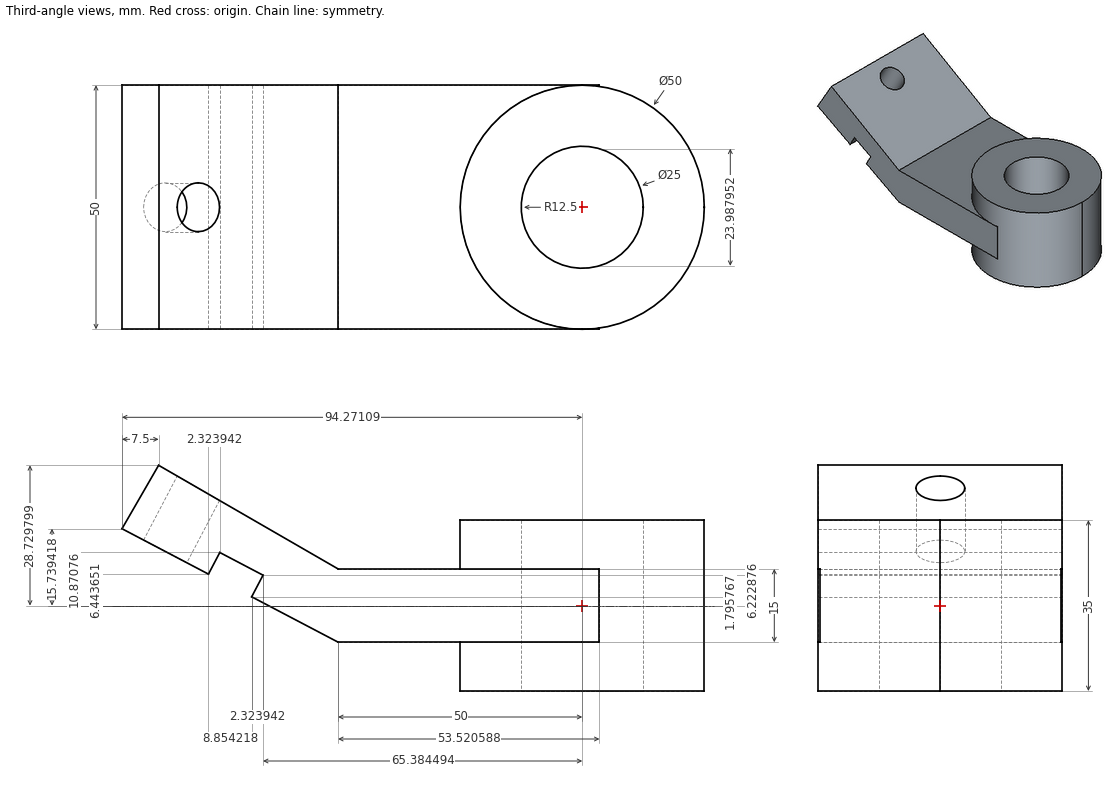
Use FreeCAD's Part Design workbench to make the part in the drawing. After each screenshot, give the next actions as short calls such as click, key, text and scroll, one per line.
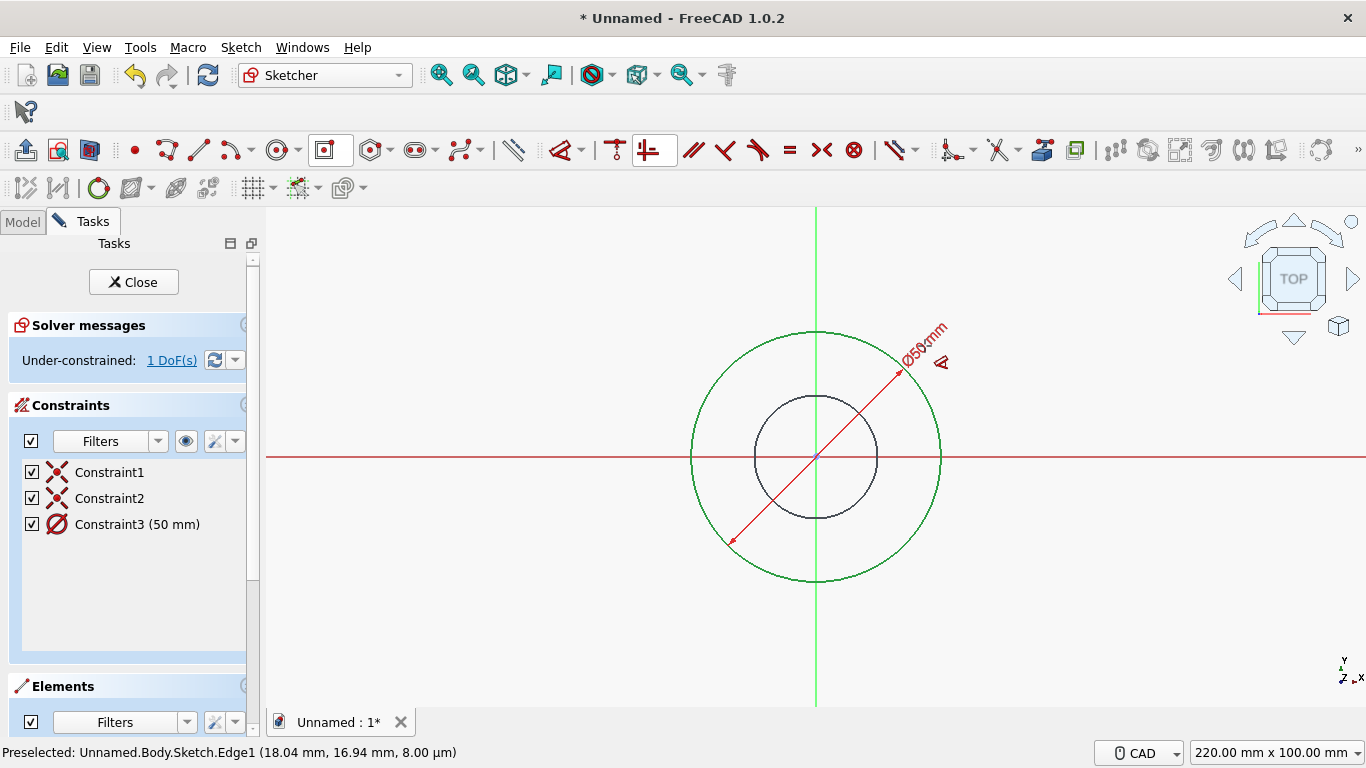
click(859, 413)
click(881, 390)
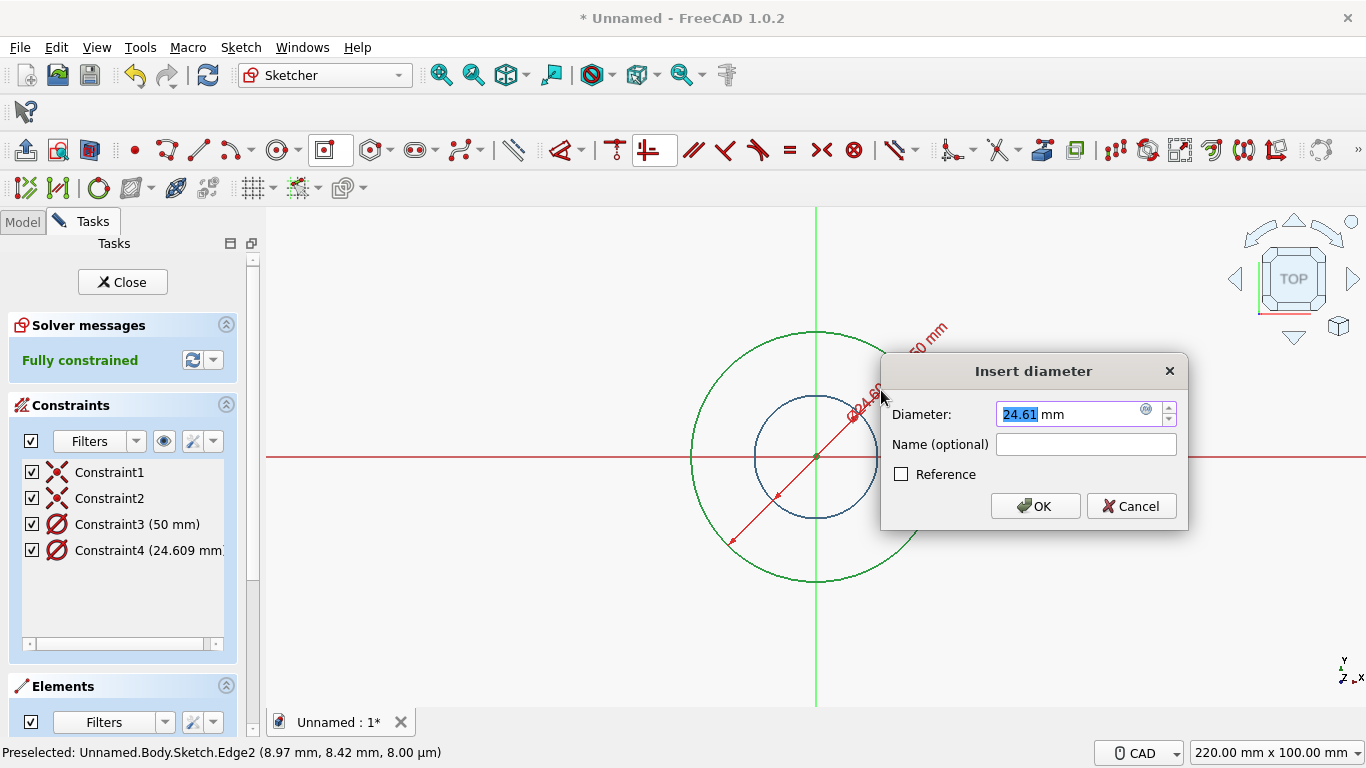
text(25)
key(Return)
key(Escape)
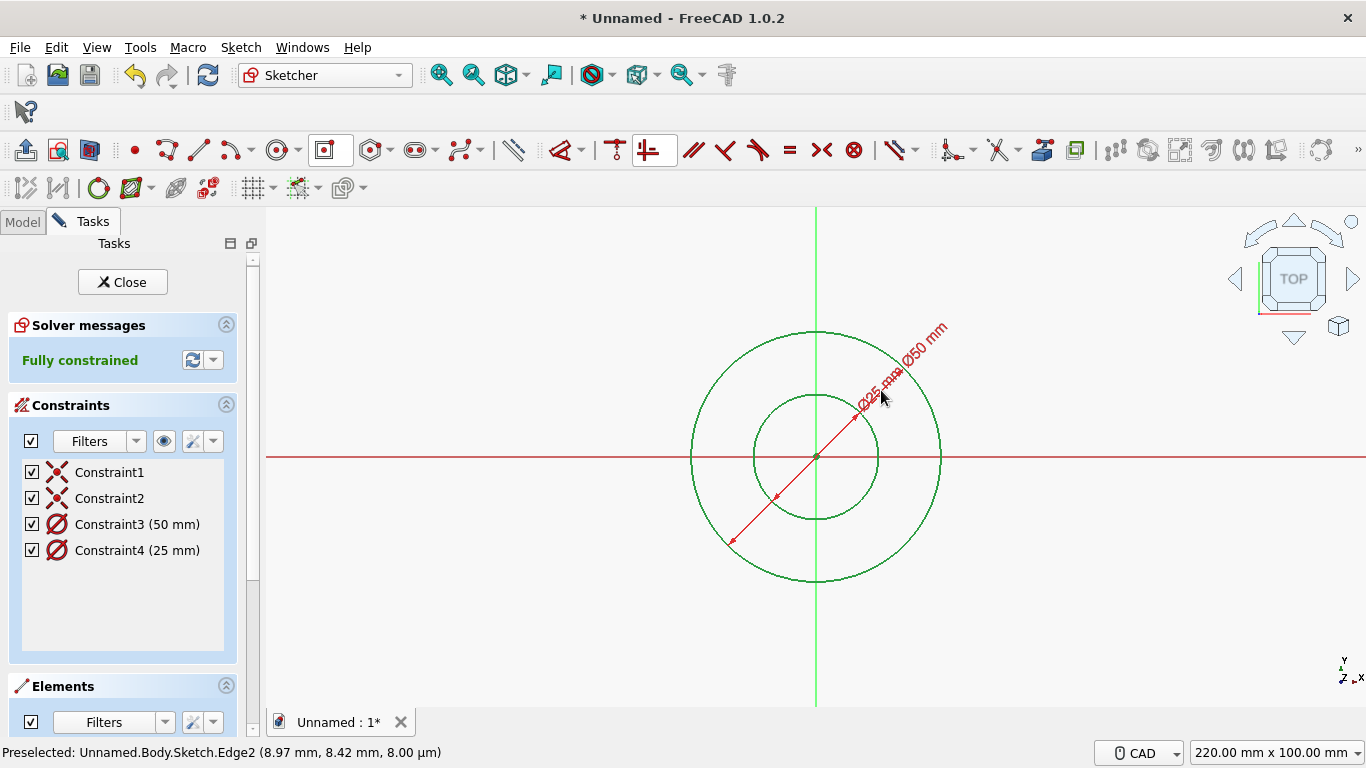
click(123, 282)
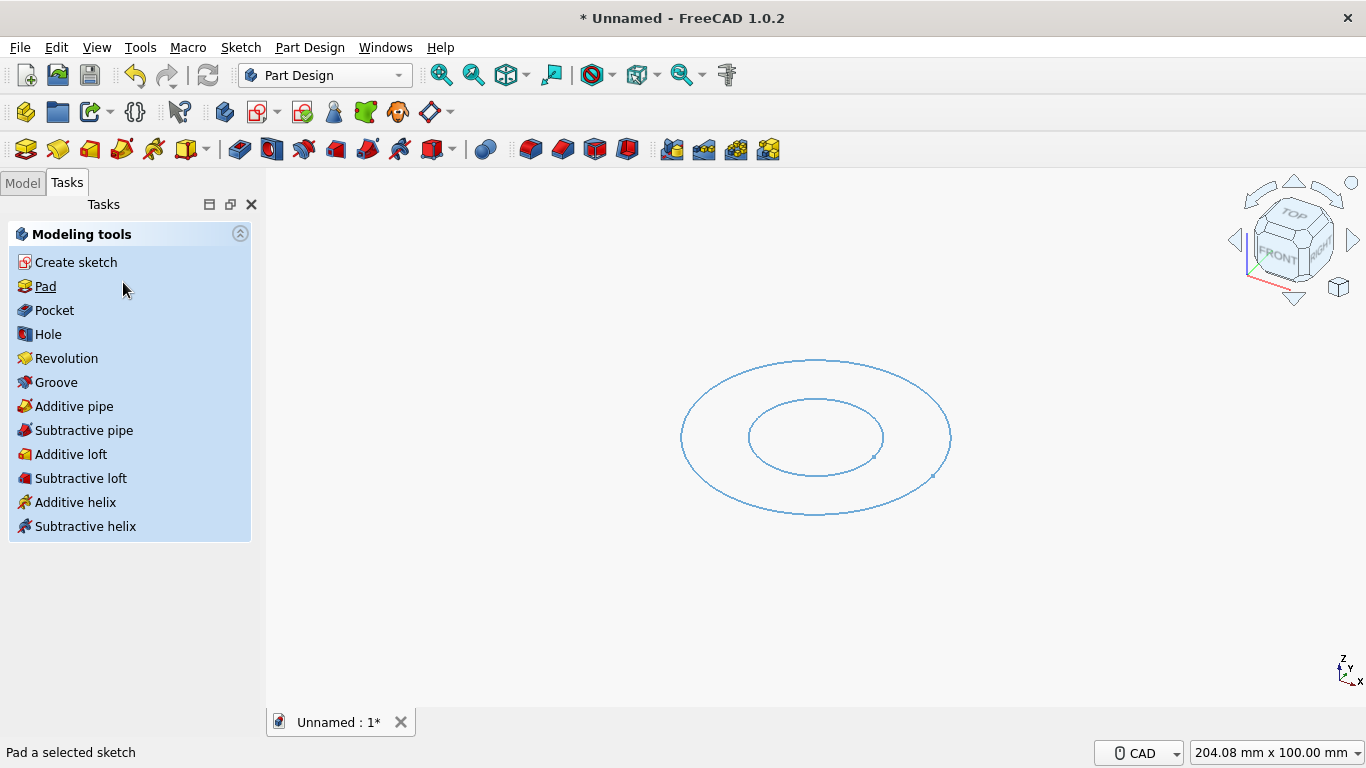
click(26, 150)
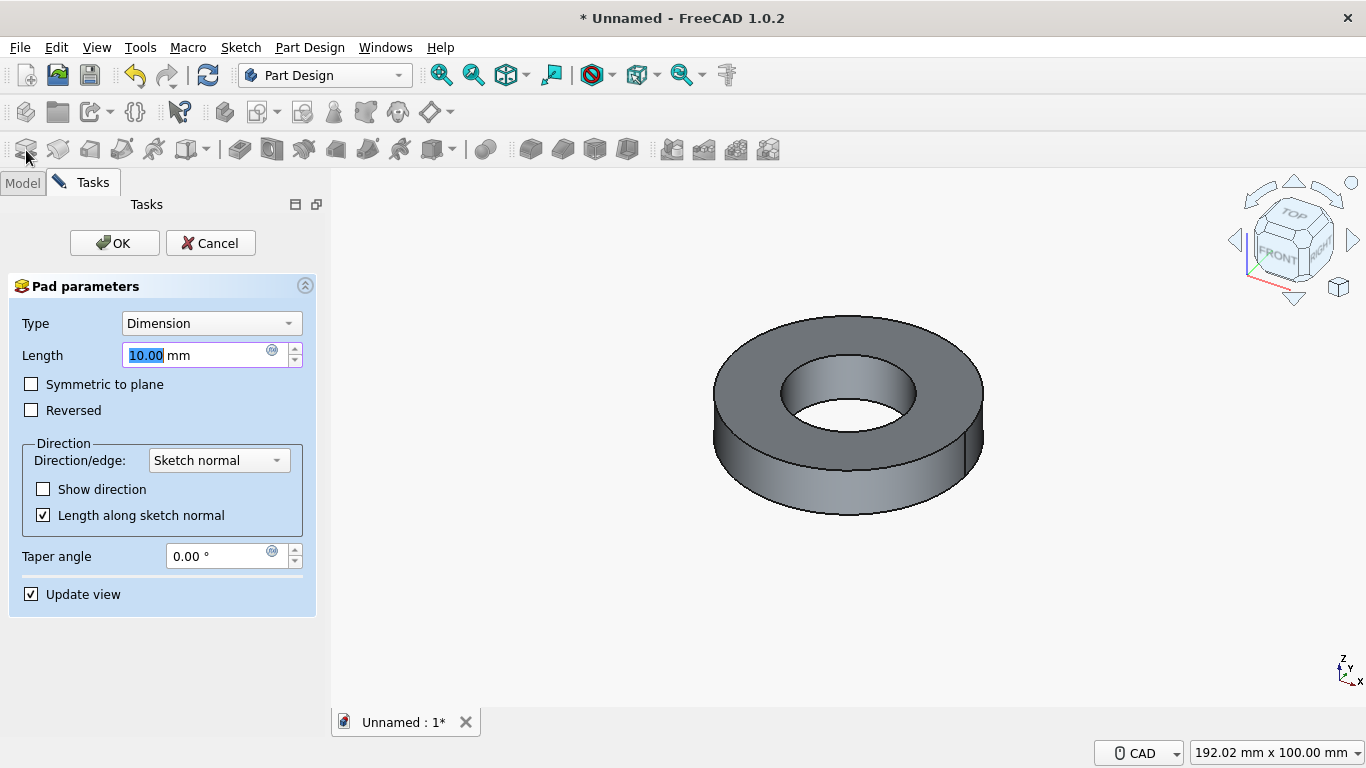
text(35)
key(Tab)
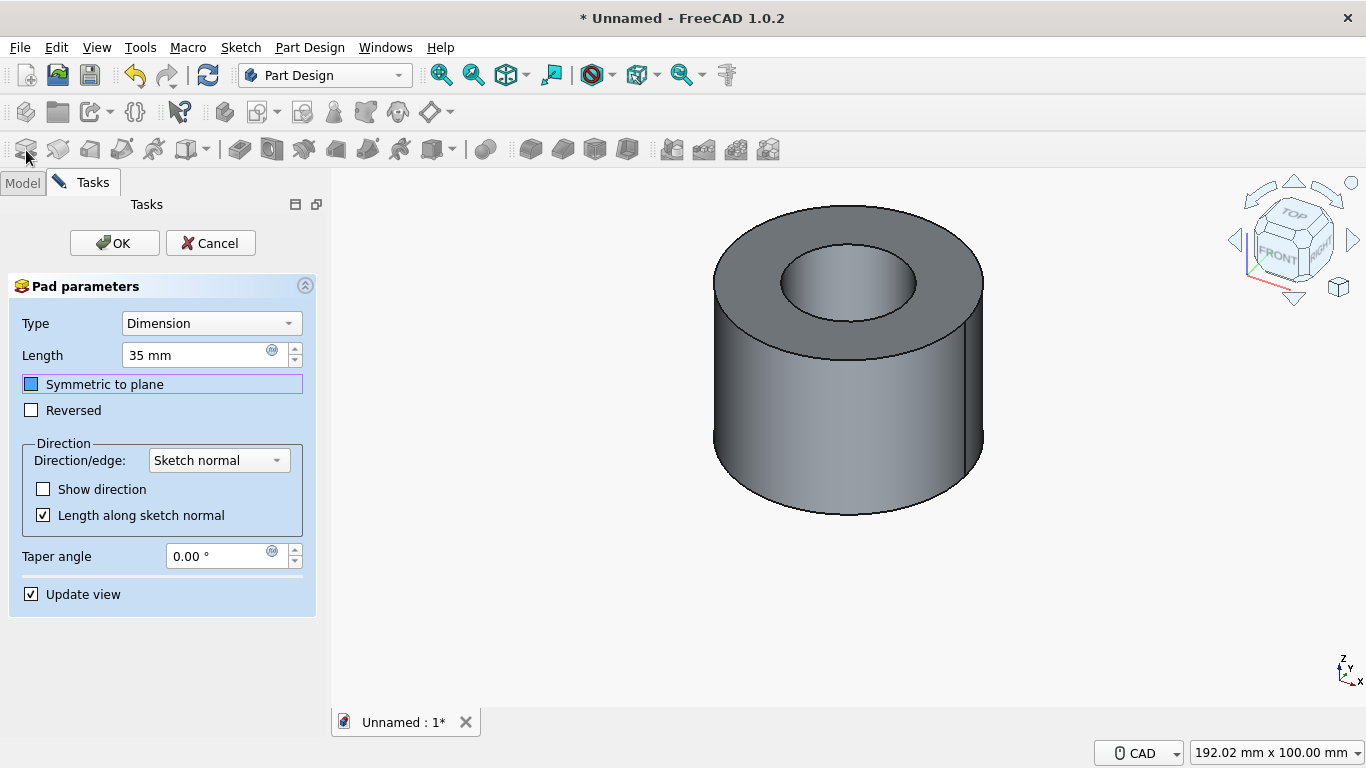
click(30, 384)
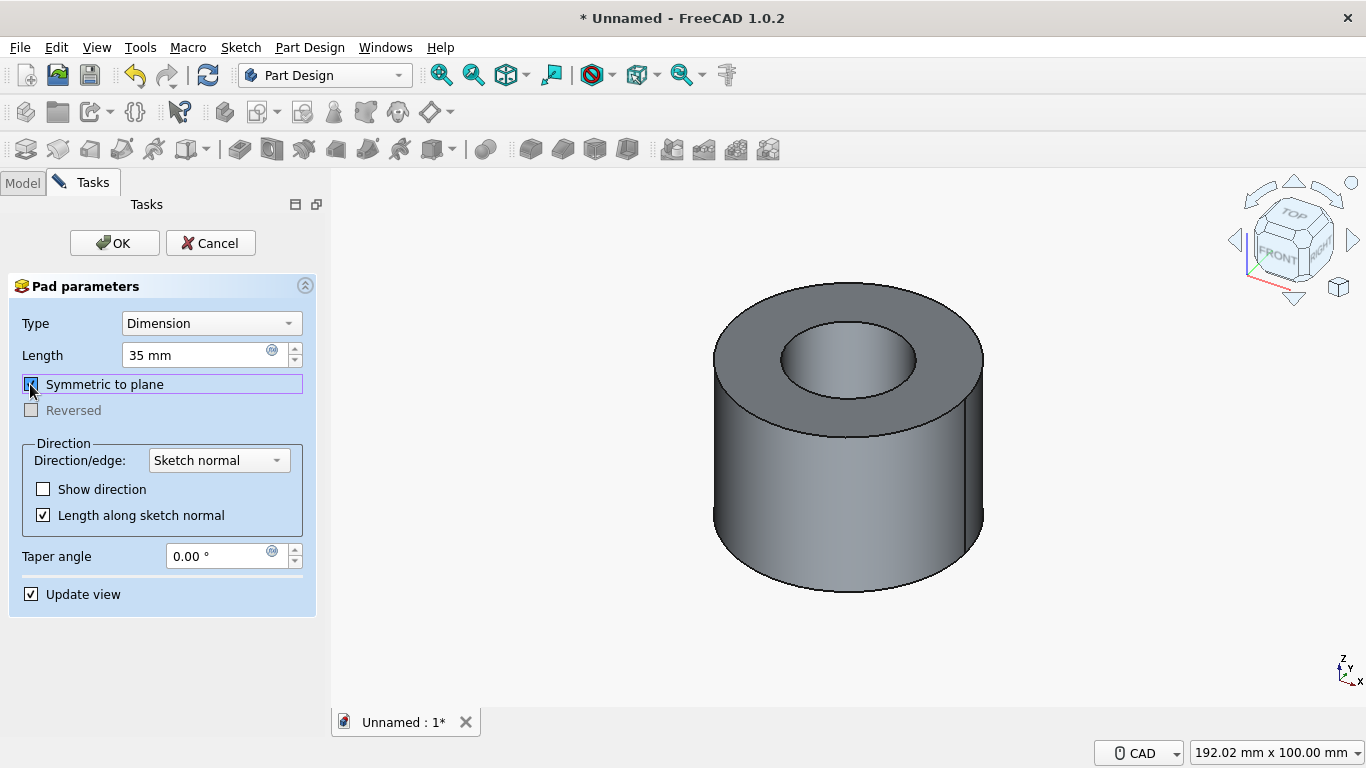
click(115, 243)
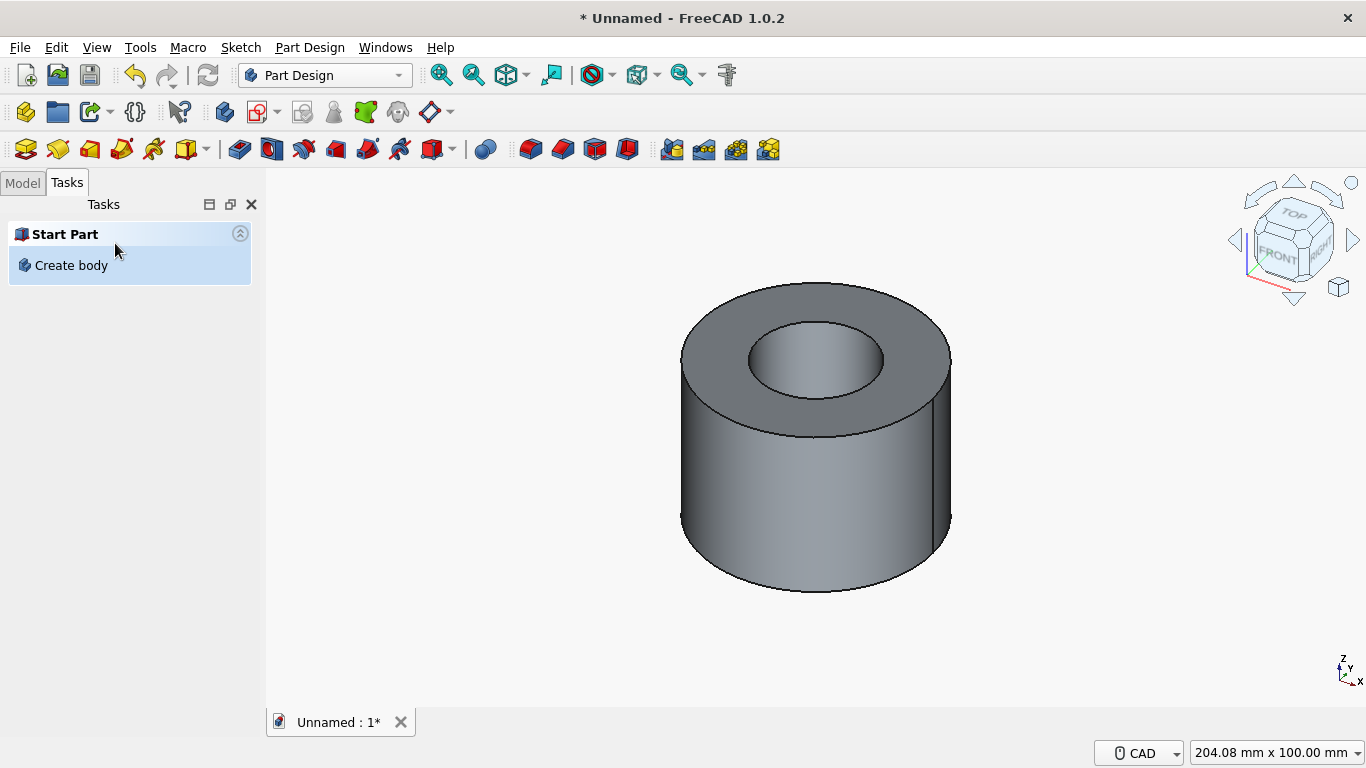
click(258, 112)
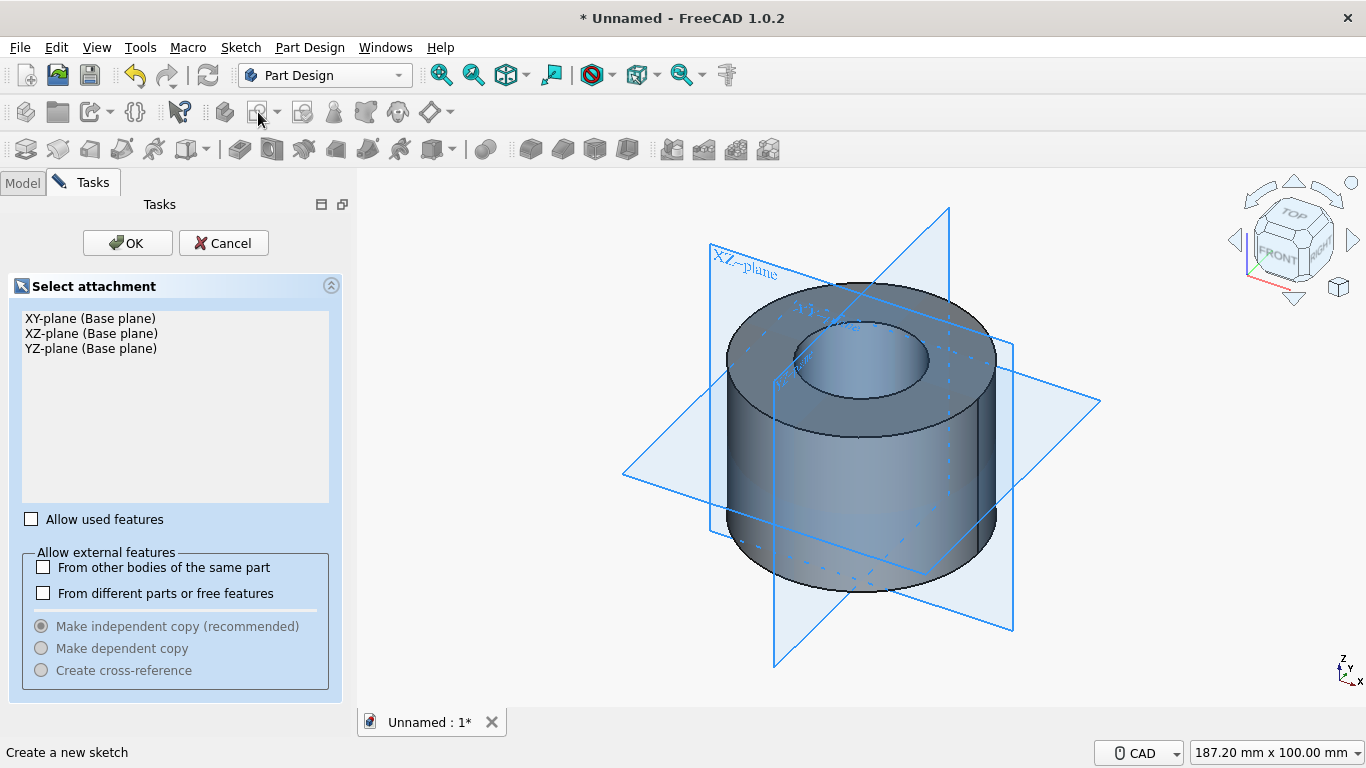
click(82, 334)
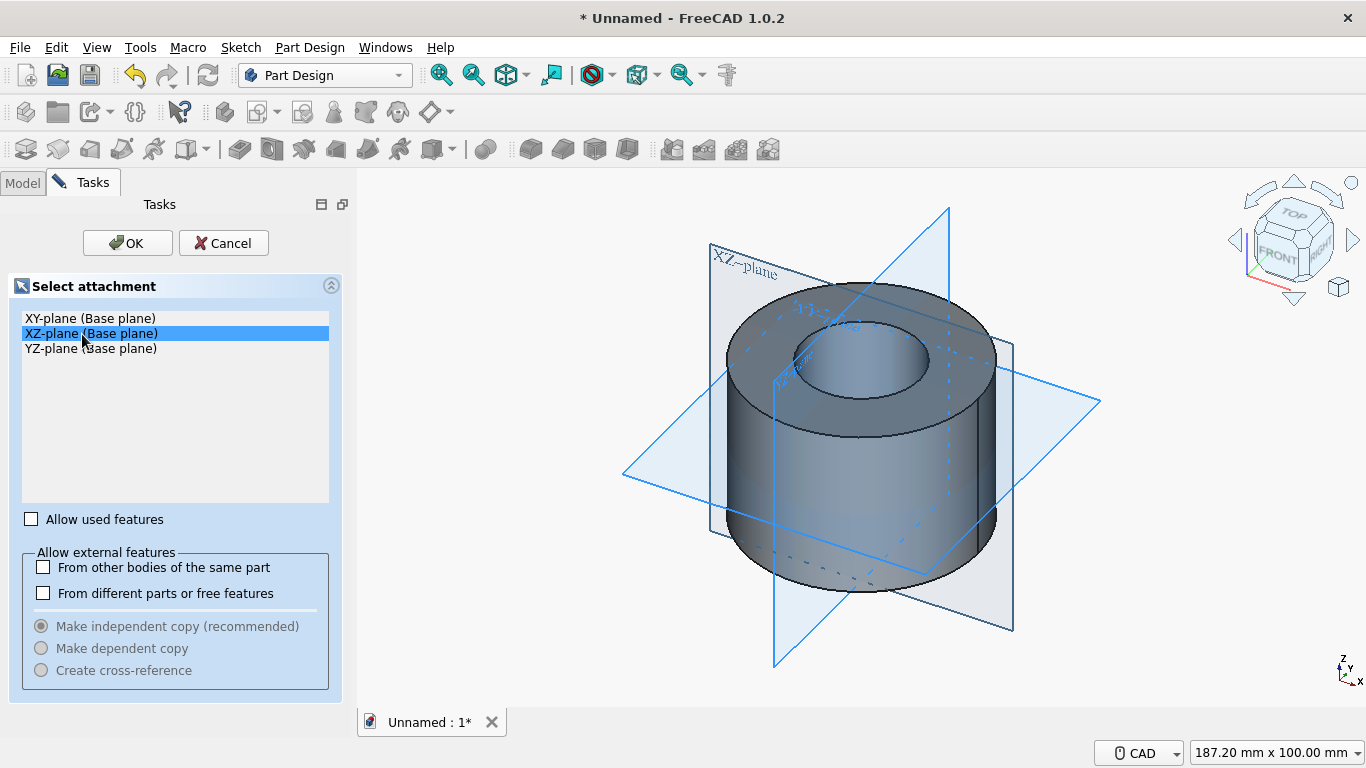
click(128, 243)